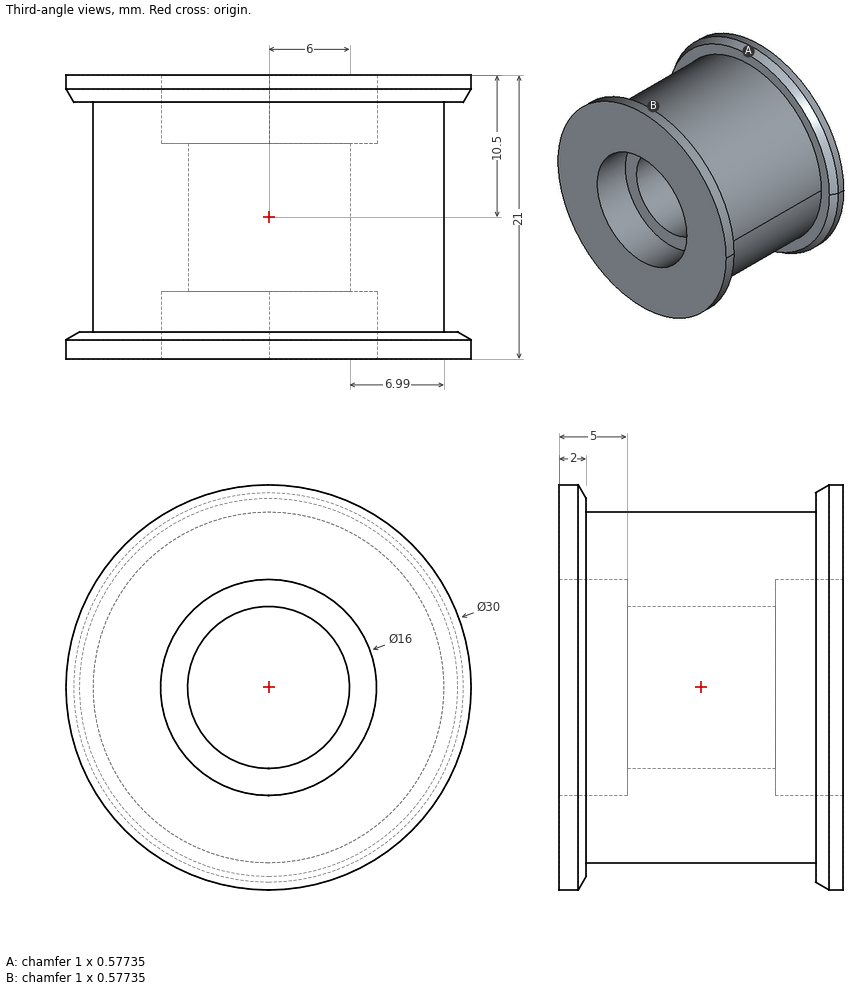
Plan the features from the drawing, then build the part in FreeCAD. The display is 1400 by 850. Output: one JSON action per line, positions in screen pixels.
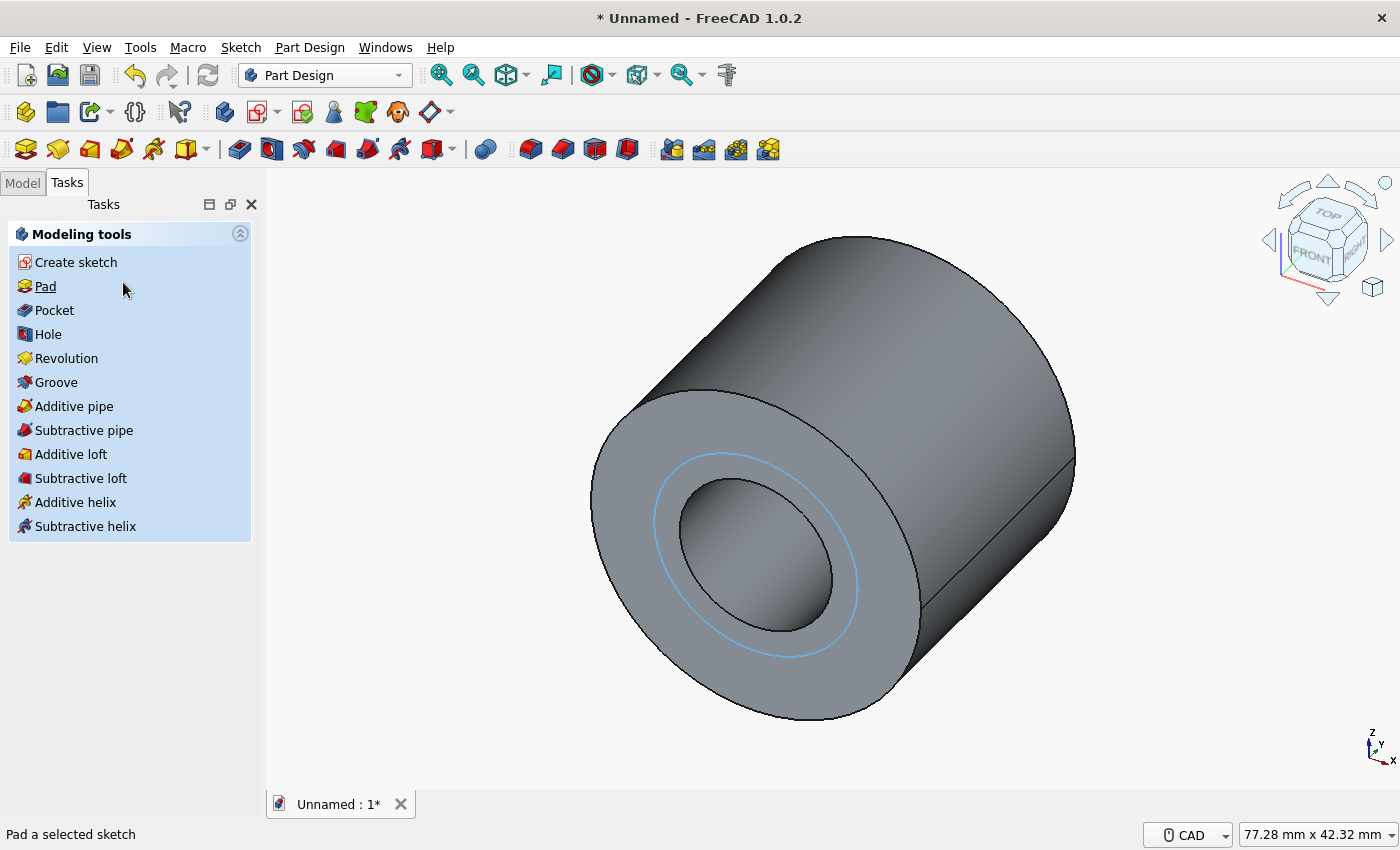
{"action": "left_click", "coordinate": [240, 150]}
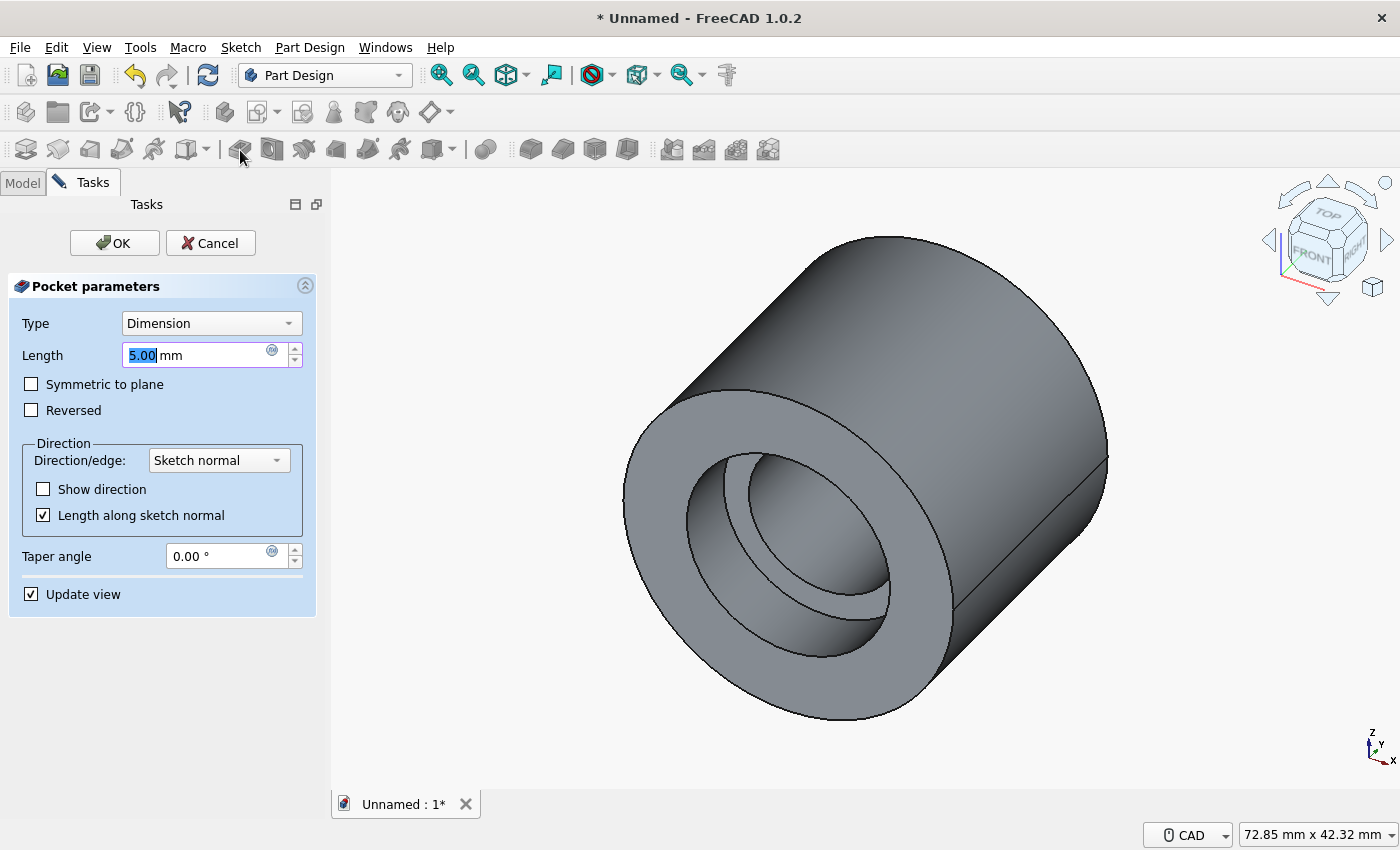
{"action": "type", "text": "5"}
{"action": "key", "text": "Tab"}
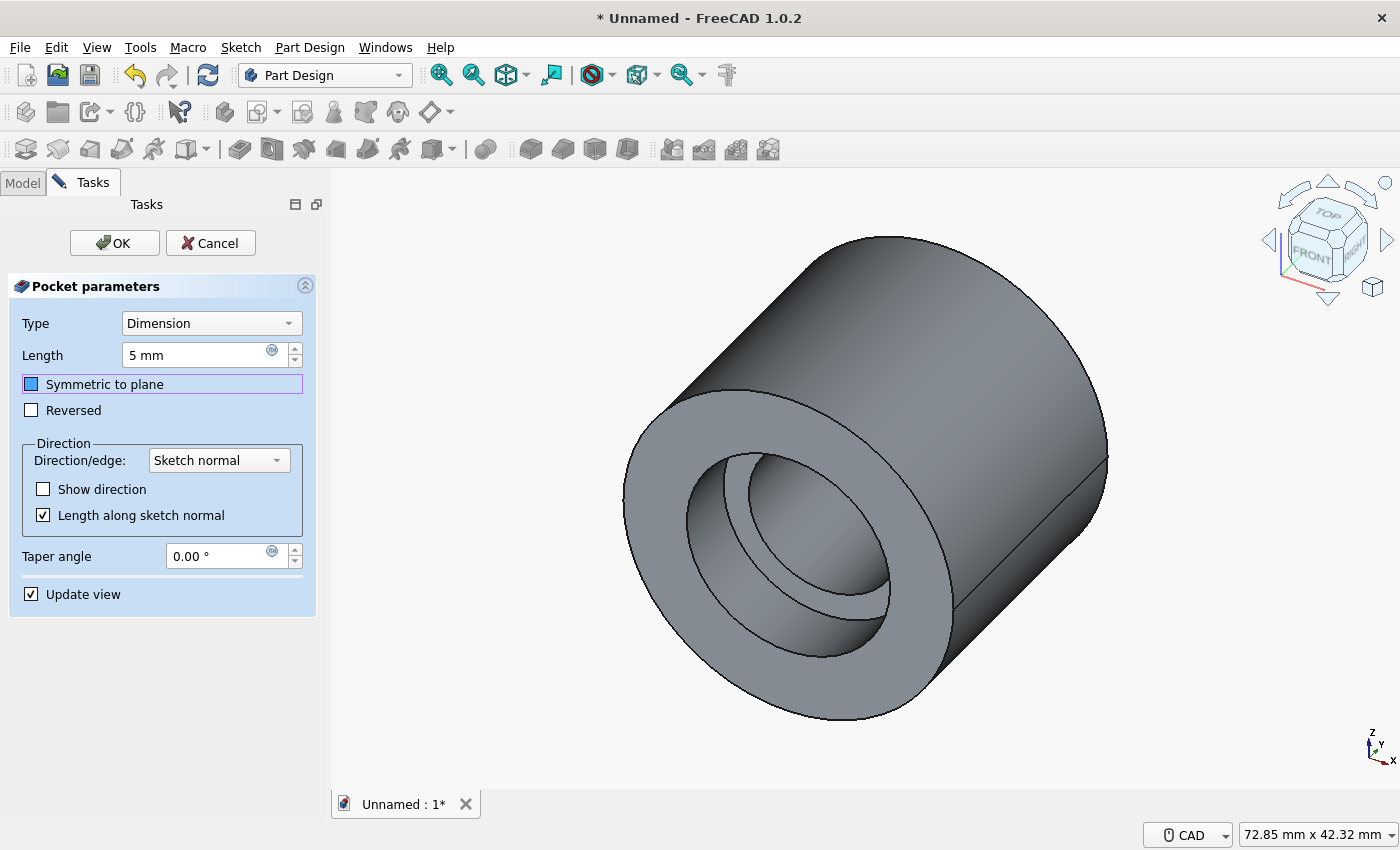
{"action": "left_click", "coordinate": [115, 243]}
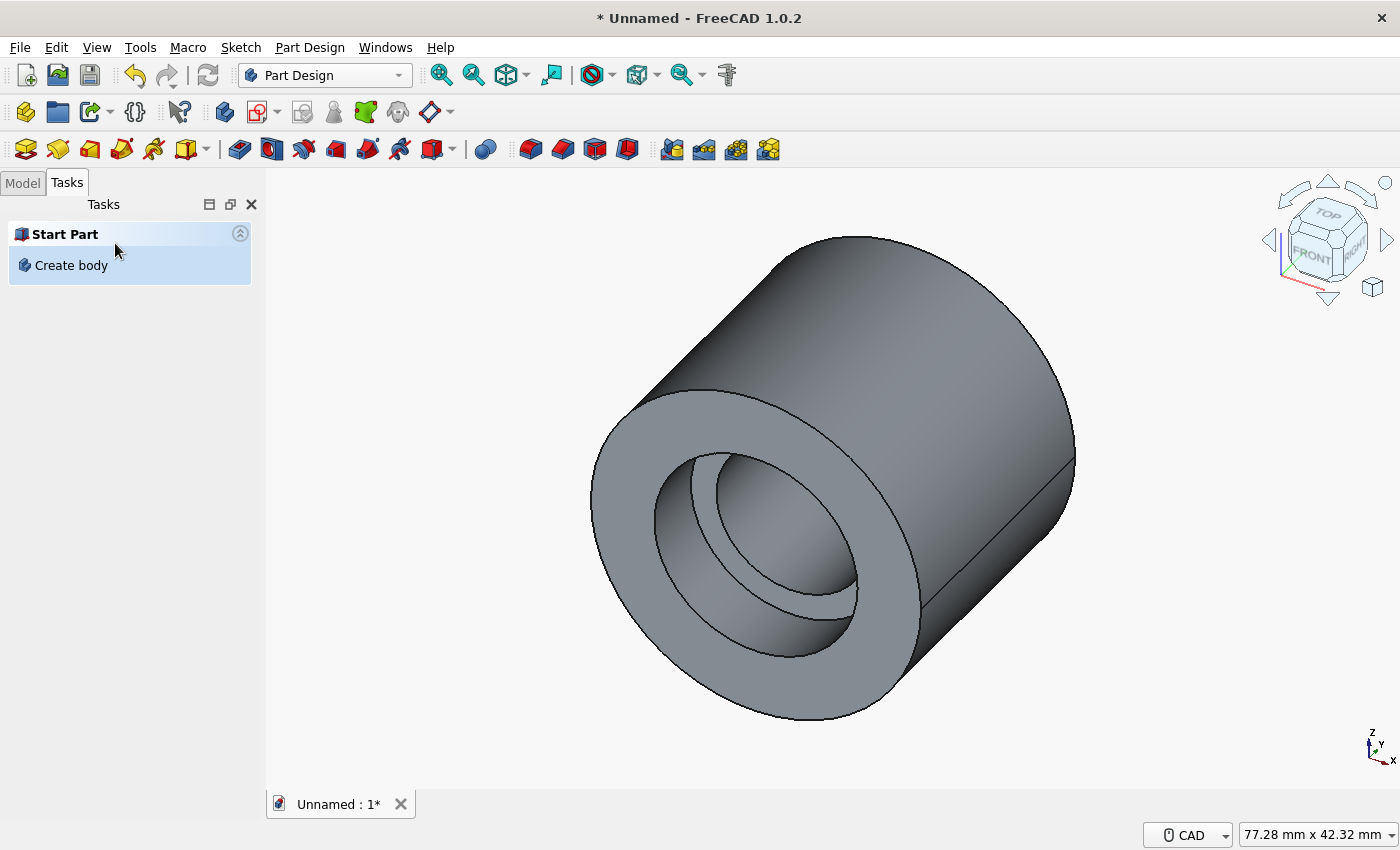
{"action": "left_click", "coordinate": [850, 674]}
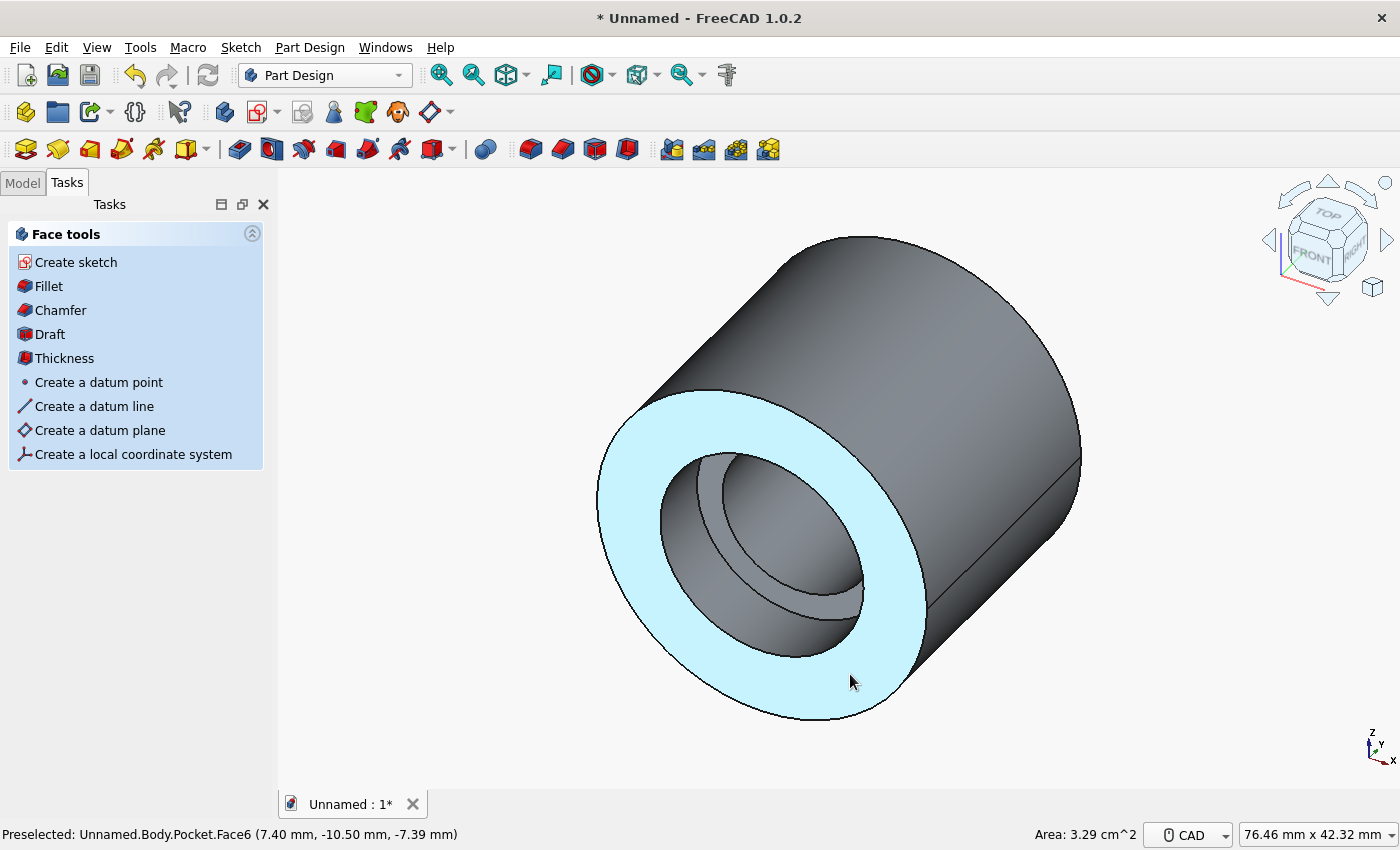
{"action": "left_click", "coordinate": [258, 112]}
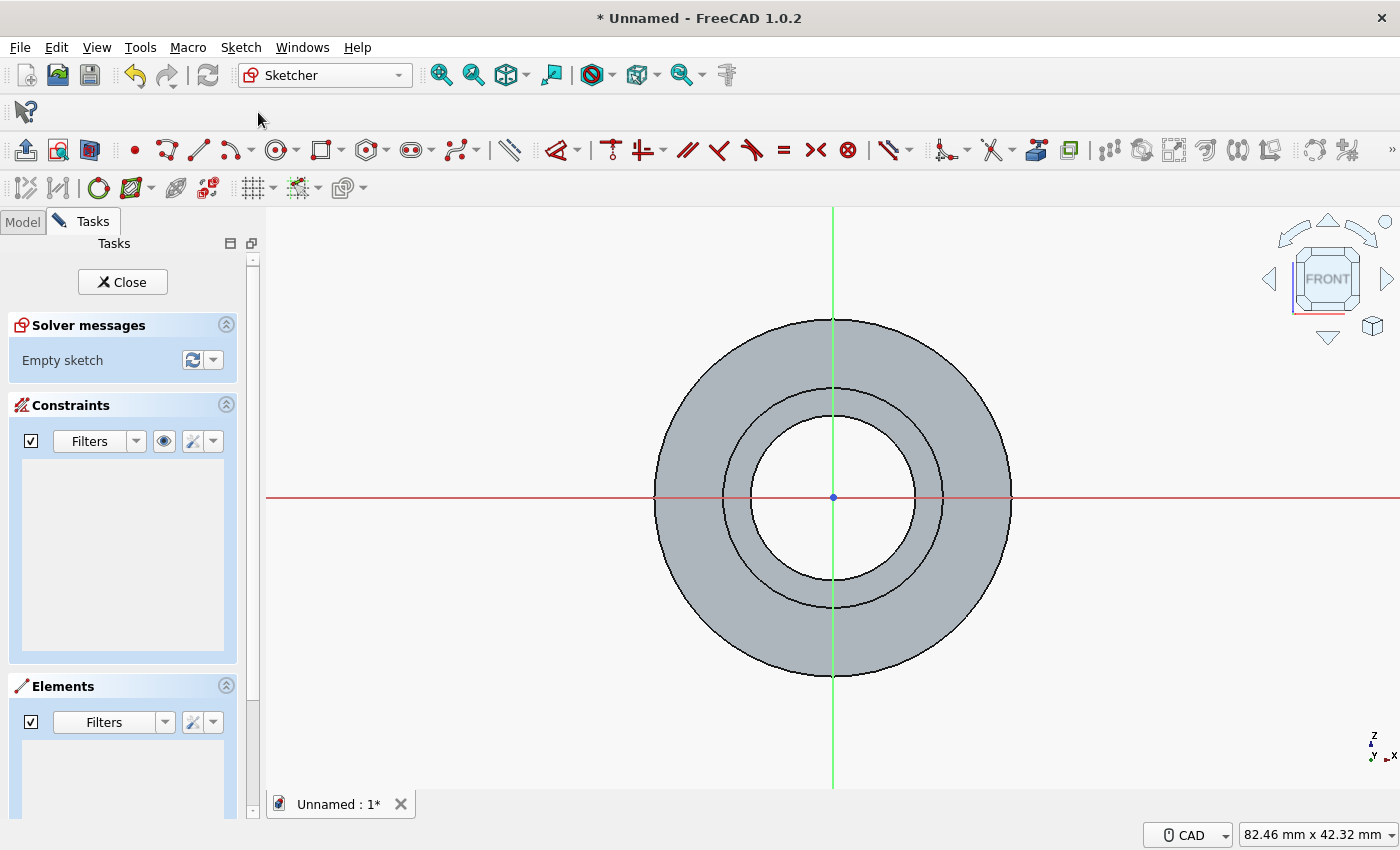
{"action": "left_click", "coordinate": [276, 150]}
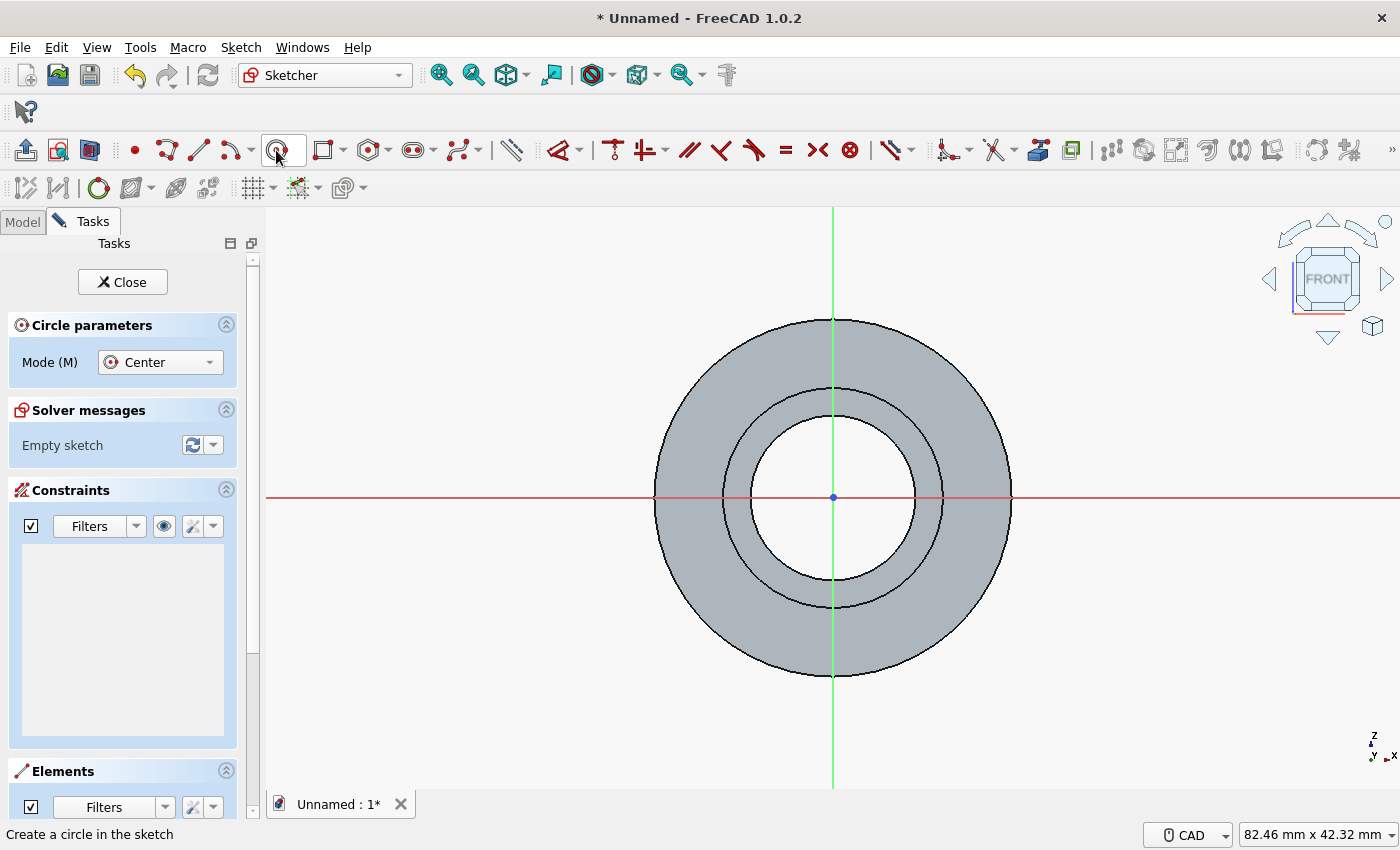
{"action": "left_click", "coordinate": [833, 498]}
{"action": "mouse_move", "coordinate": [979, 352]}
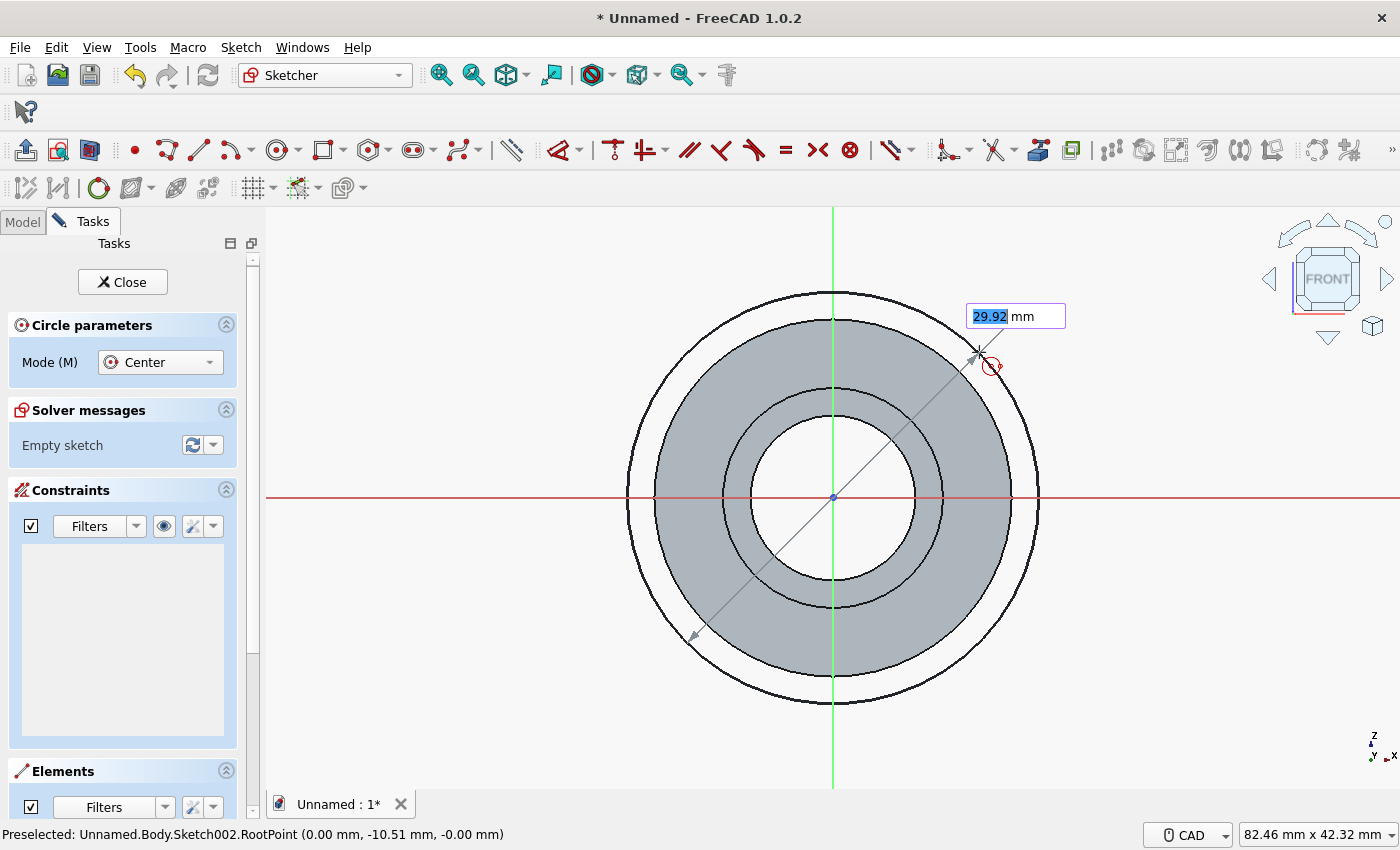
{"action": "type", "text": "30"}
{"action": "key", "text": "Return"}